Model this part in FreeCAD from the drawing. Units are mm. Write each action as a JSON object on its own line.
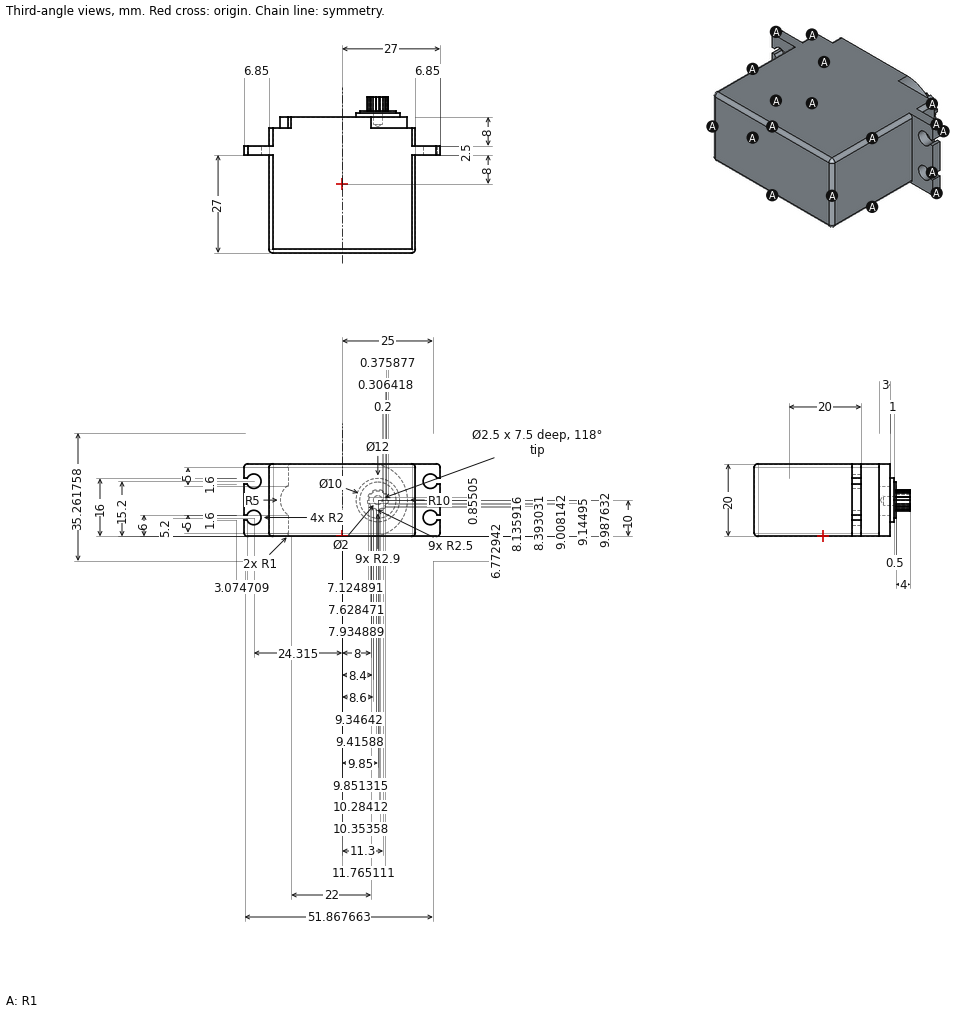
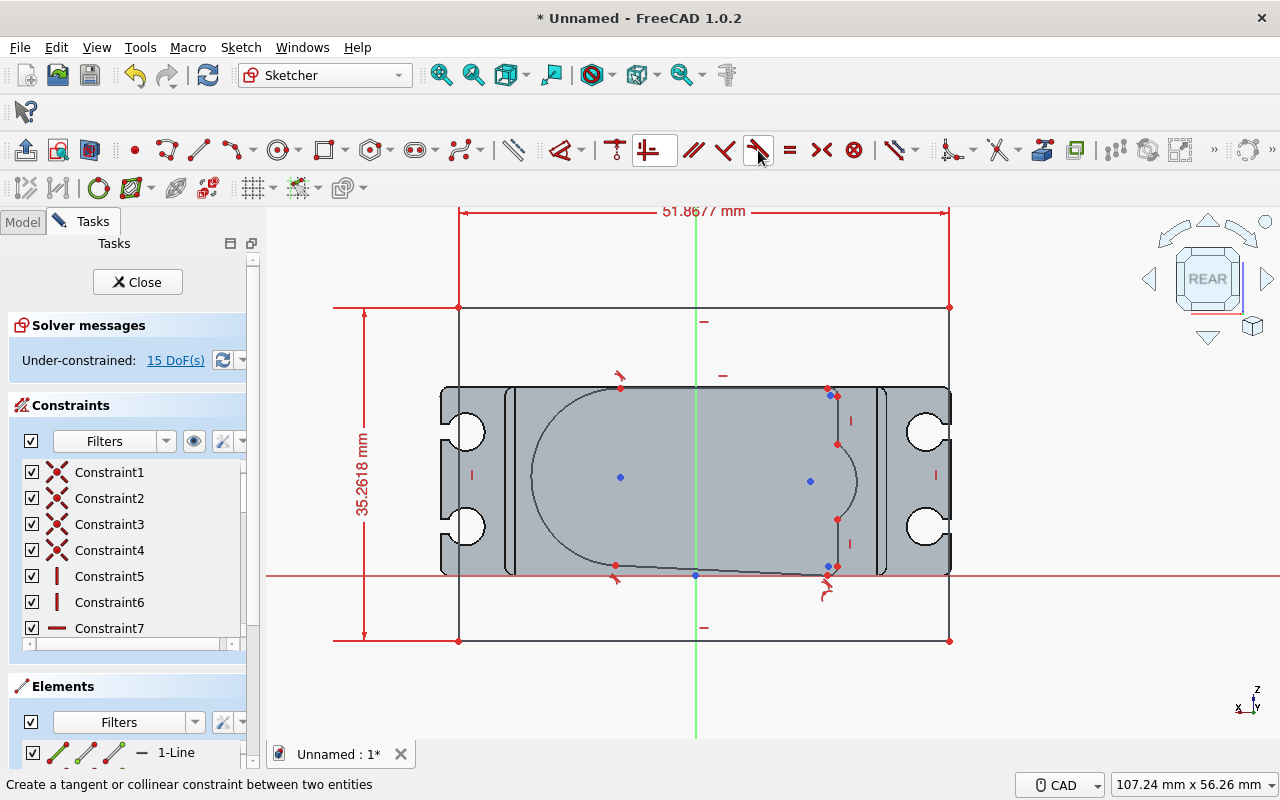
{"action": "left_click", "coordinate": [682, 388]}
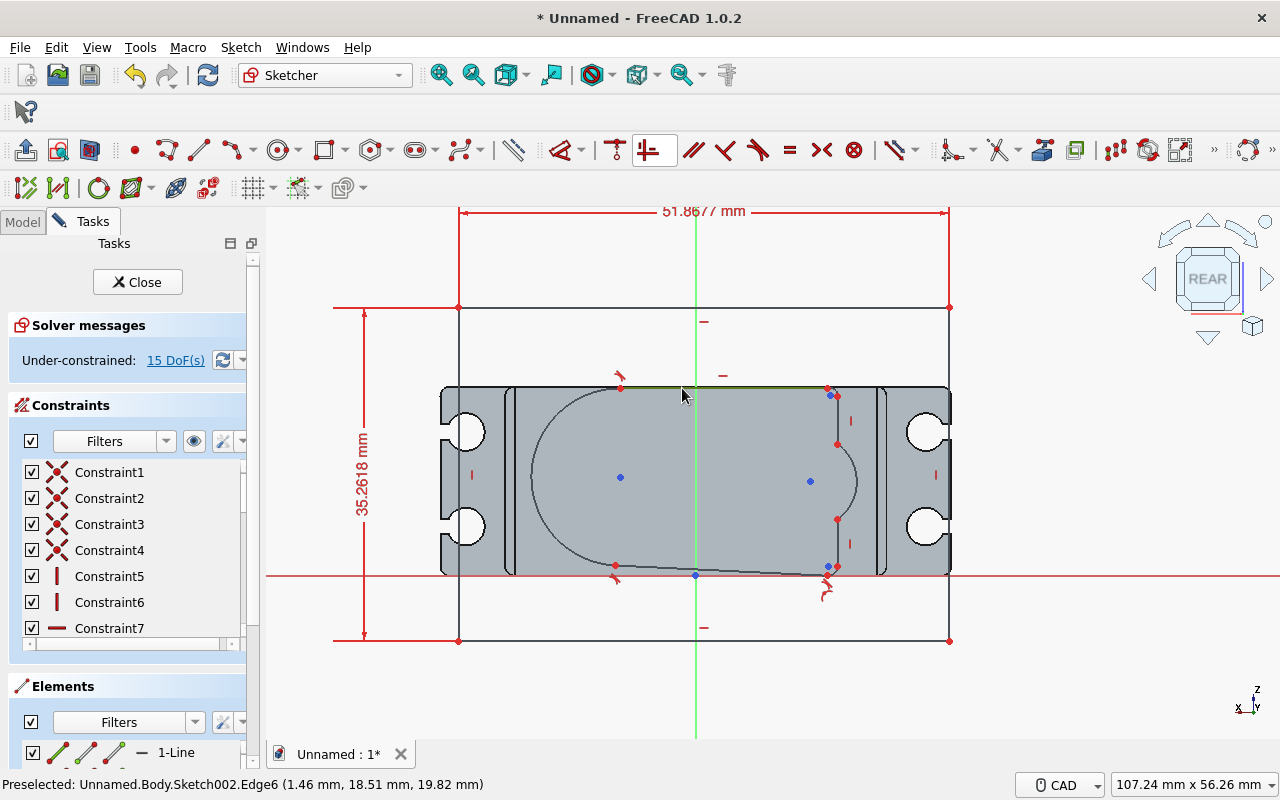
{"action": "scroll", "coordinate": [835, 390], "scroll_direction": "up", "scroll_amount": 4}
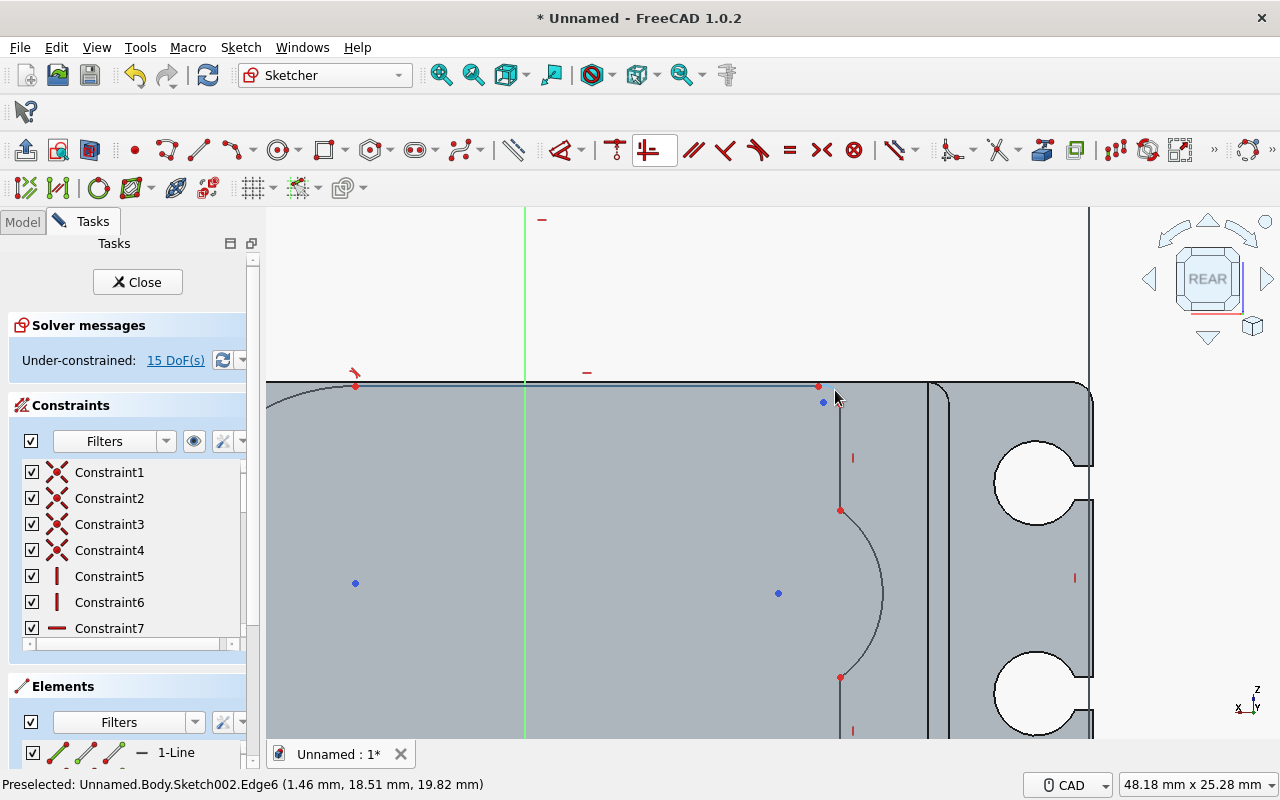
{"action": "left_click", "coordinate": [834, 389]}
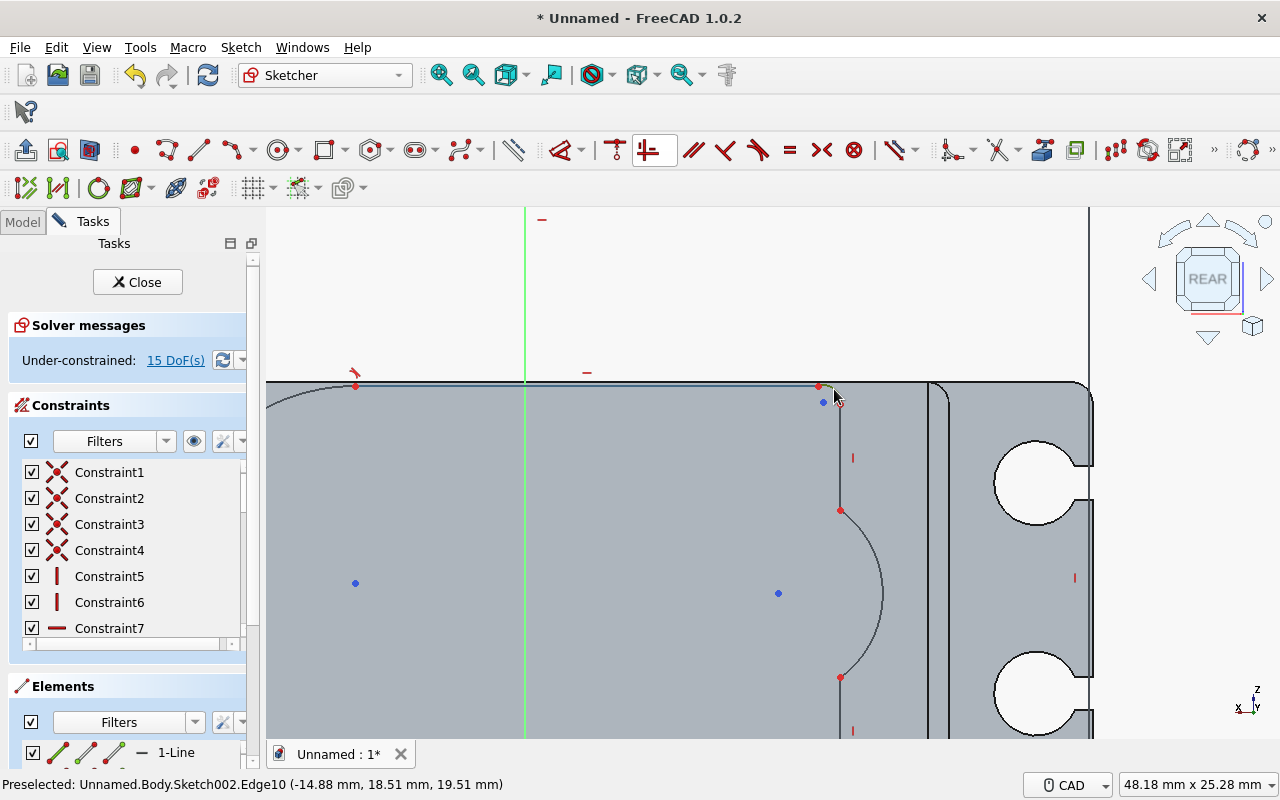
{"action": "key", "text": "t"}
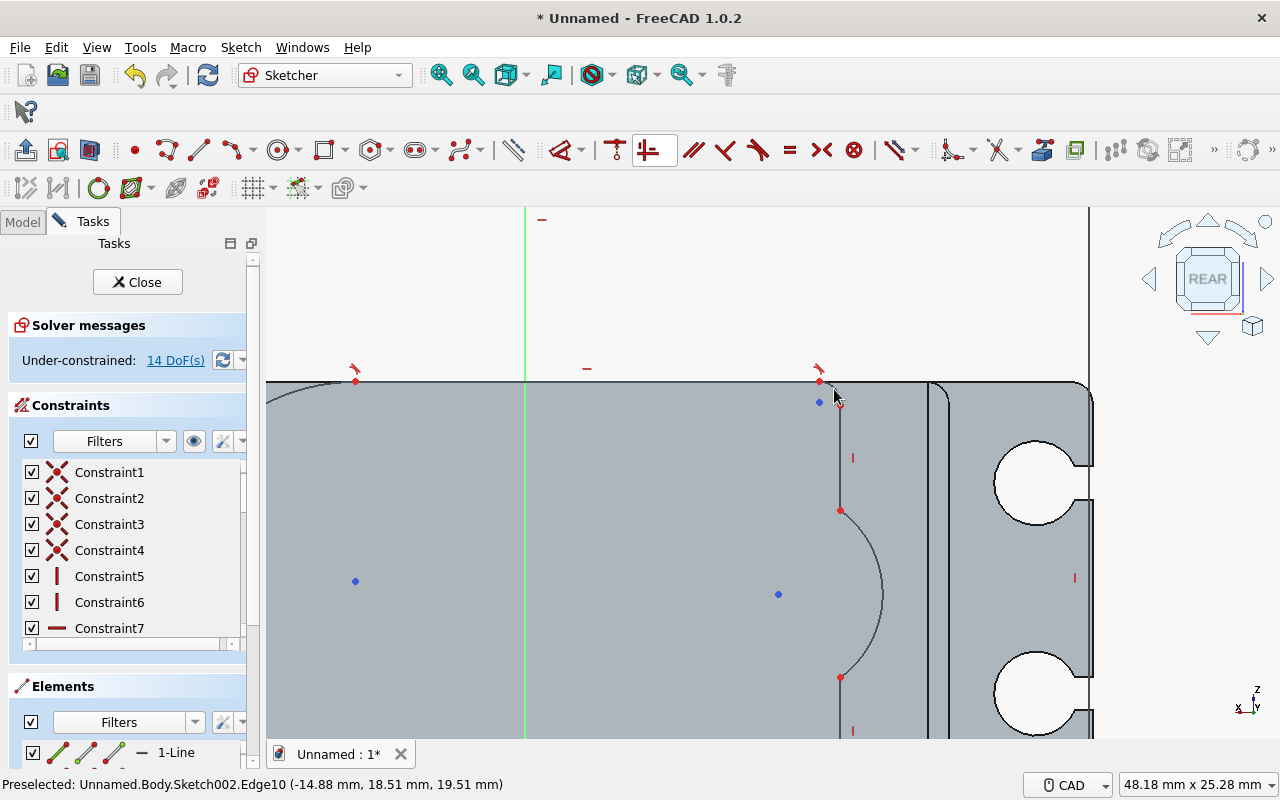
{"action": "left_click", "coordinate": [840, 437]}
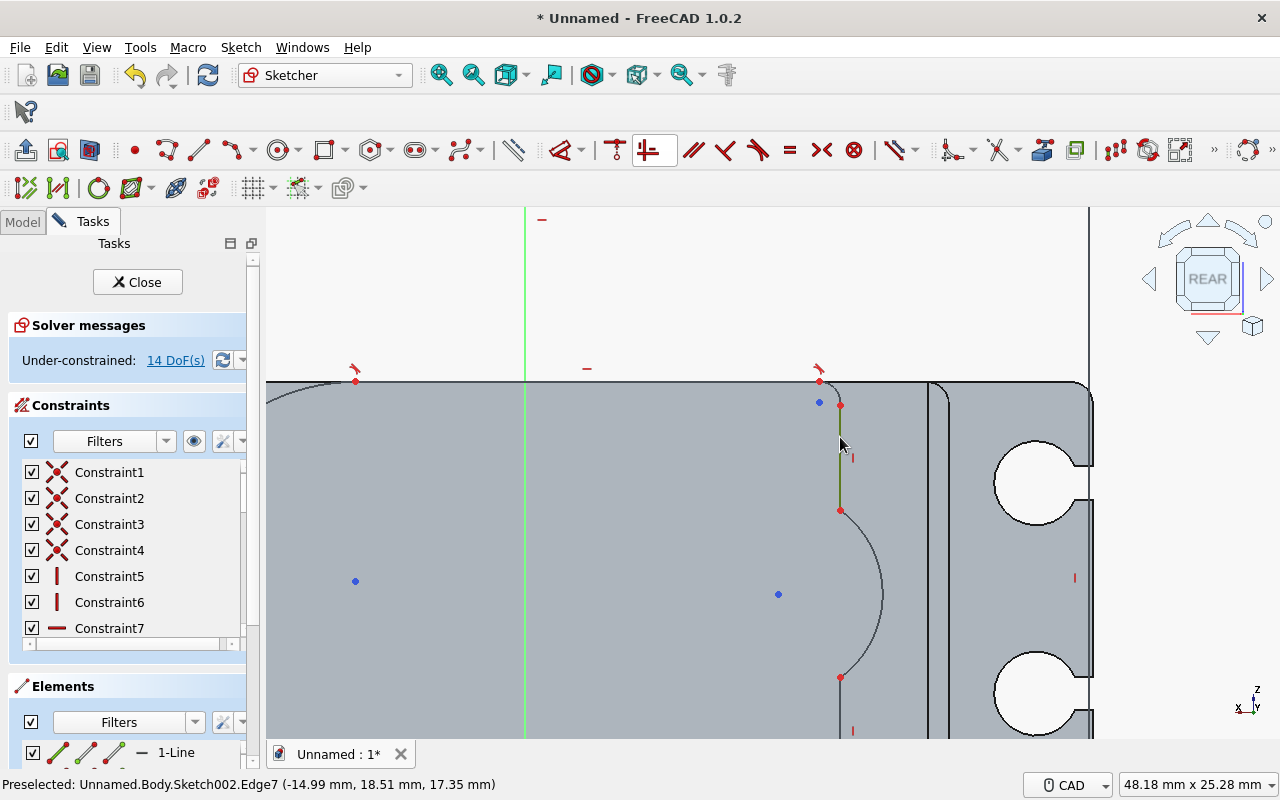
{"action": "scroll", "coordinate": [839, 395], "scroll_direction": "up", "scroll_amount": 2}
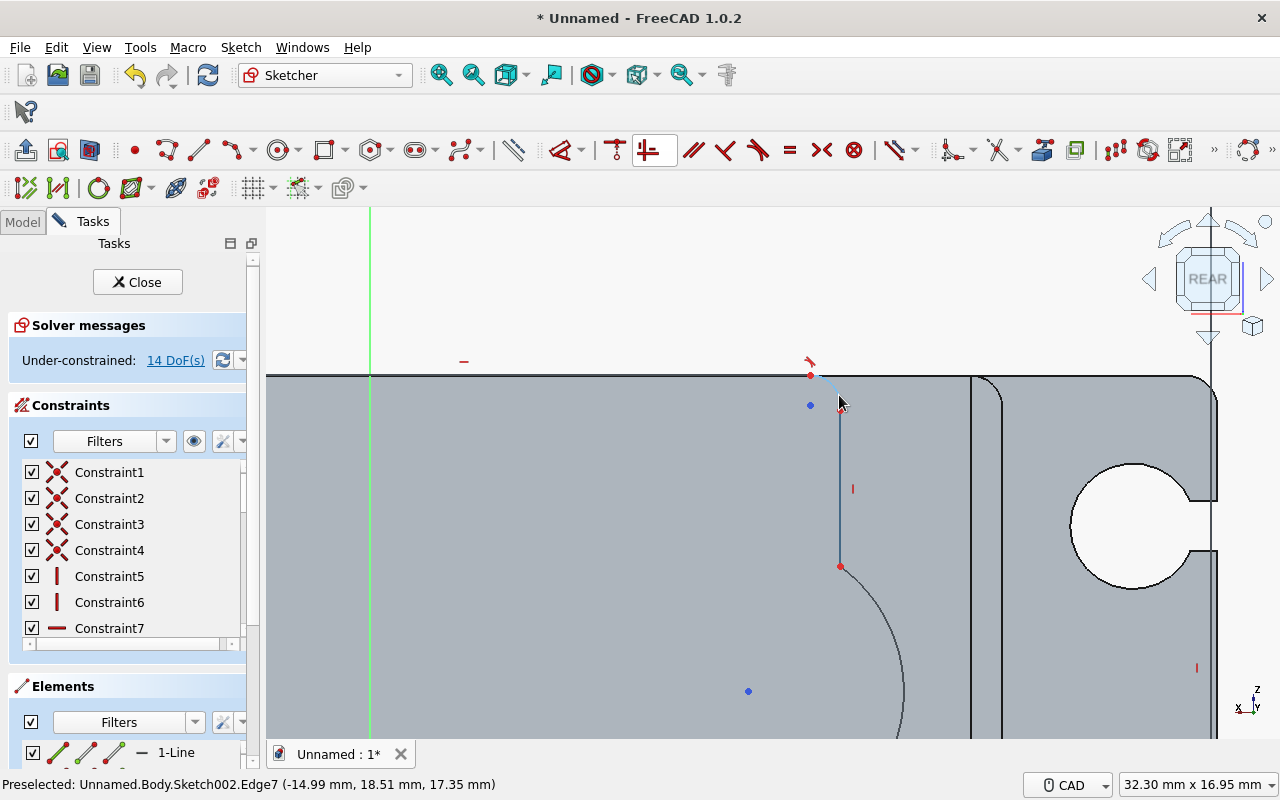
{"action": "left_click", "coordinate": [838, 395]}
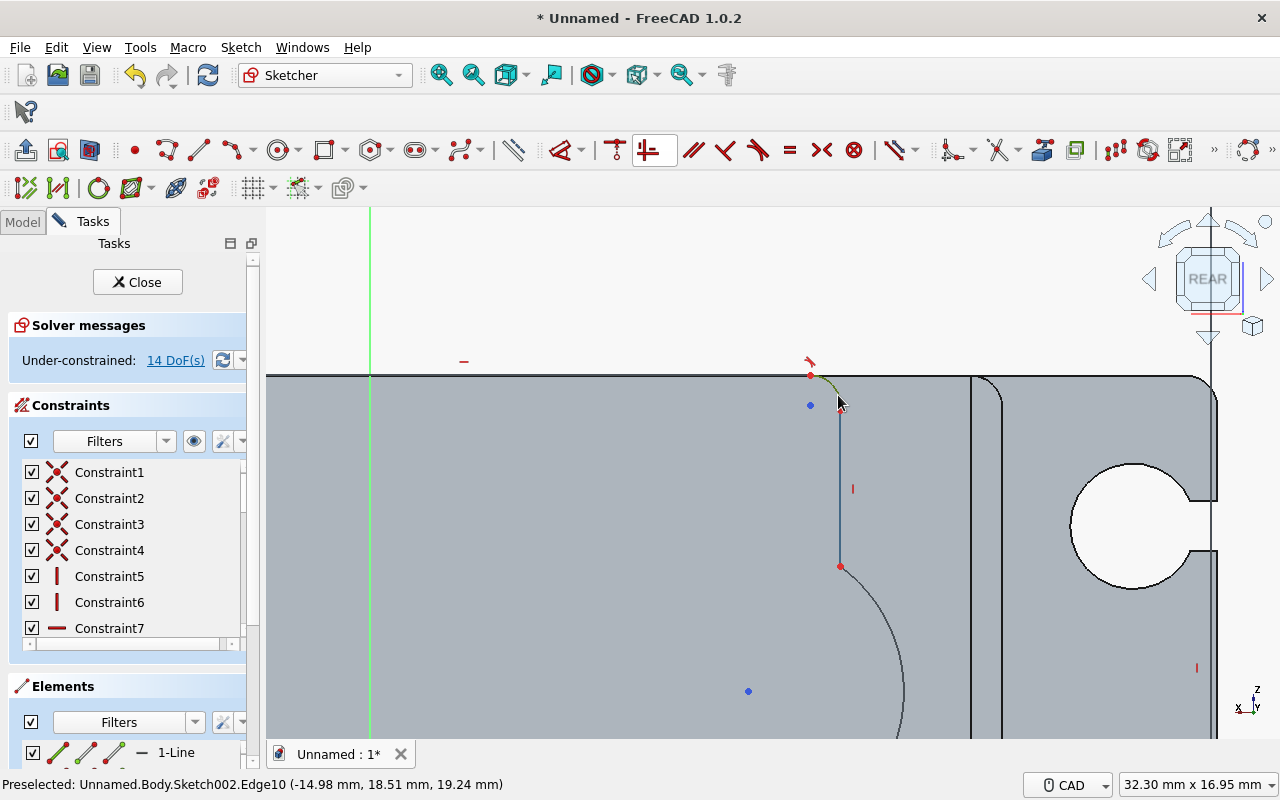
{"action": "key", "text": "t"}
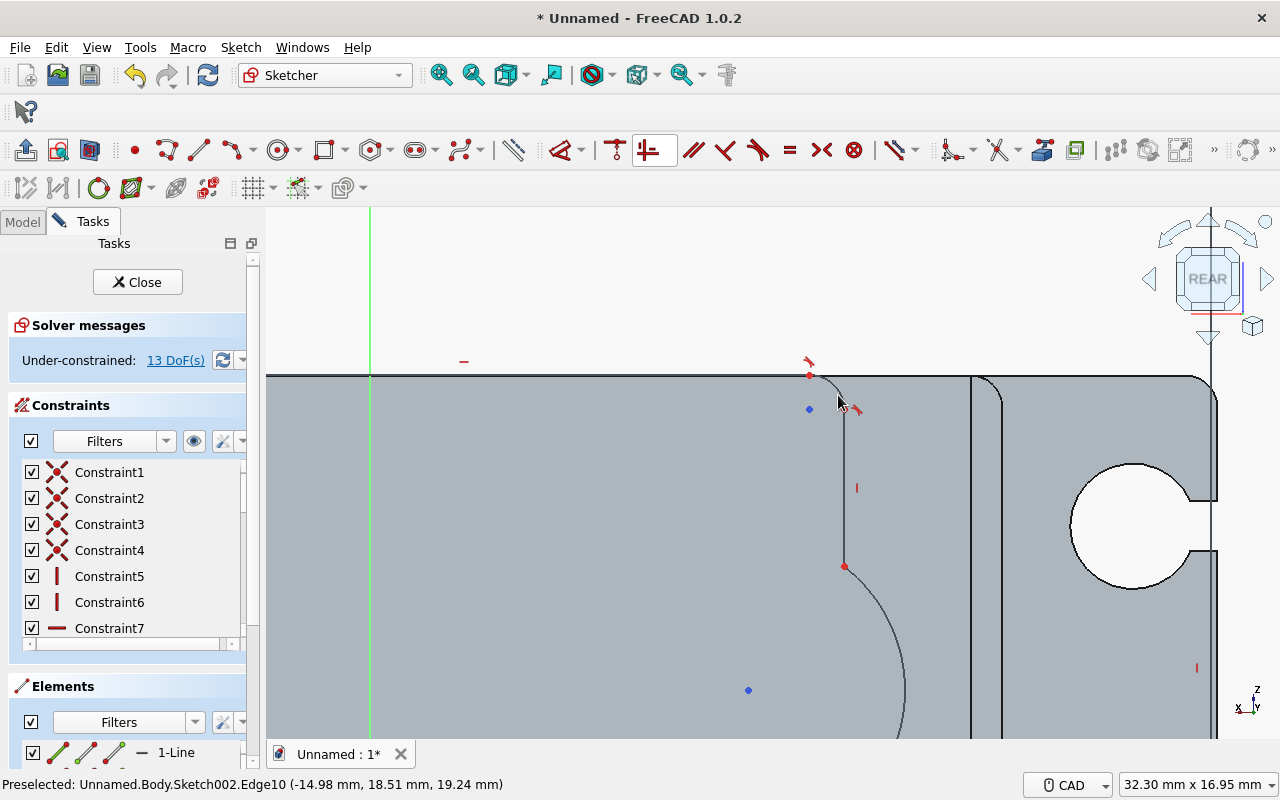
{"action": "scroll", "coordinate": [836, 391], "scroll_direction": "down", "scroll_amount": 6}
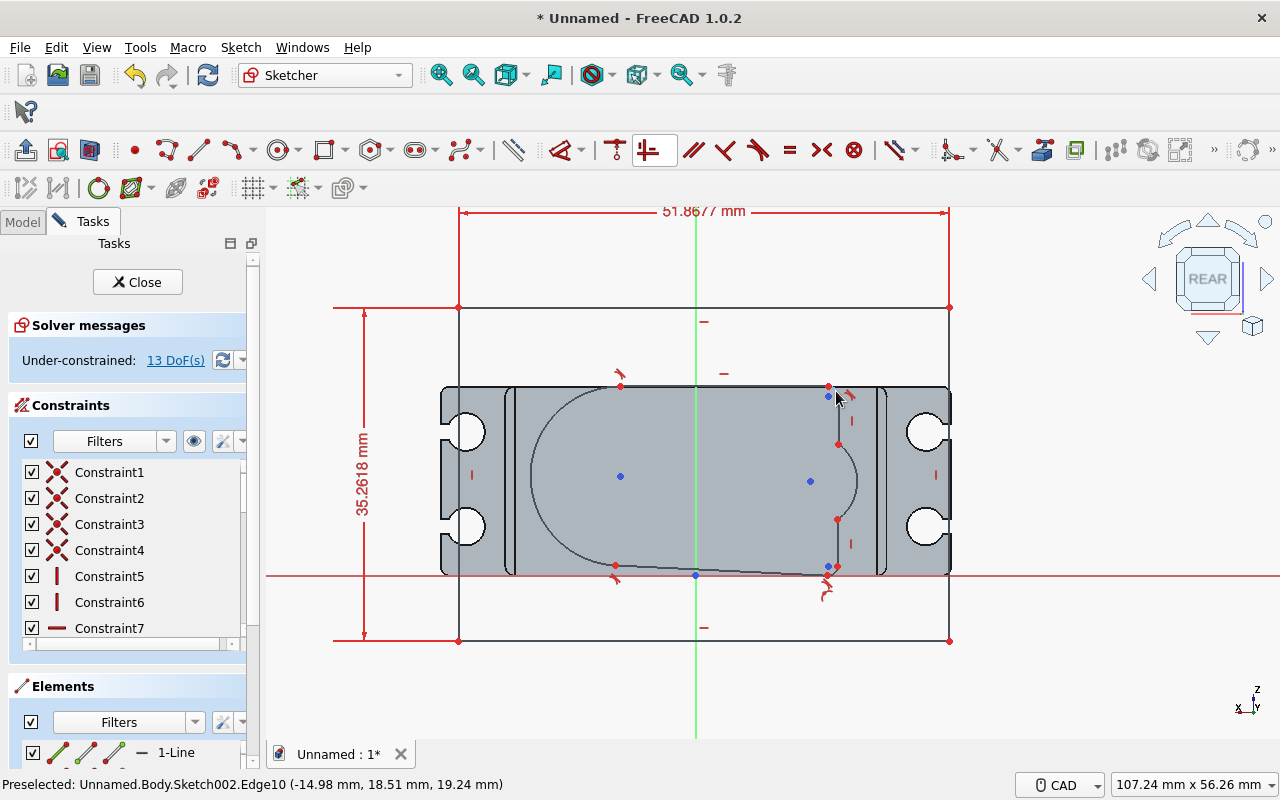
{"action": "left_click", "coordinate": [838, 534]}